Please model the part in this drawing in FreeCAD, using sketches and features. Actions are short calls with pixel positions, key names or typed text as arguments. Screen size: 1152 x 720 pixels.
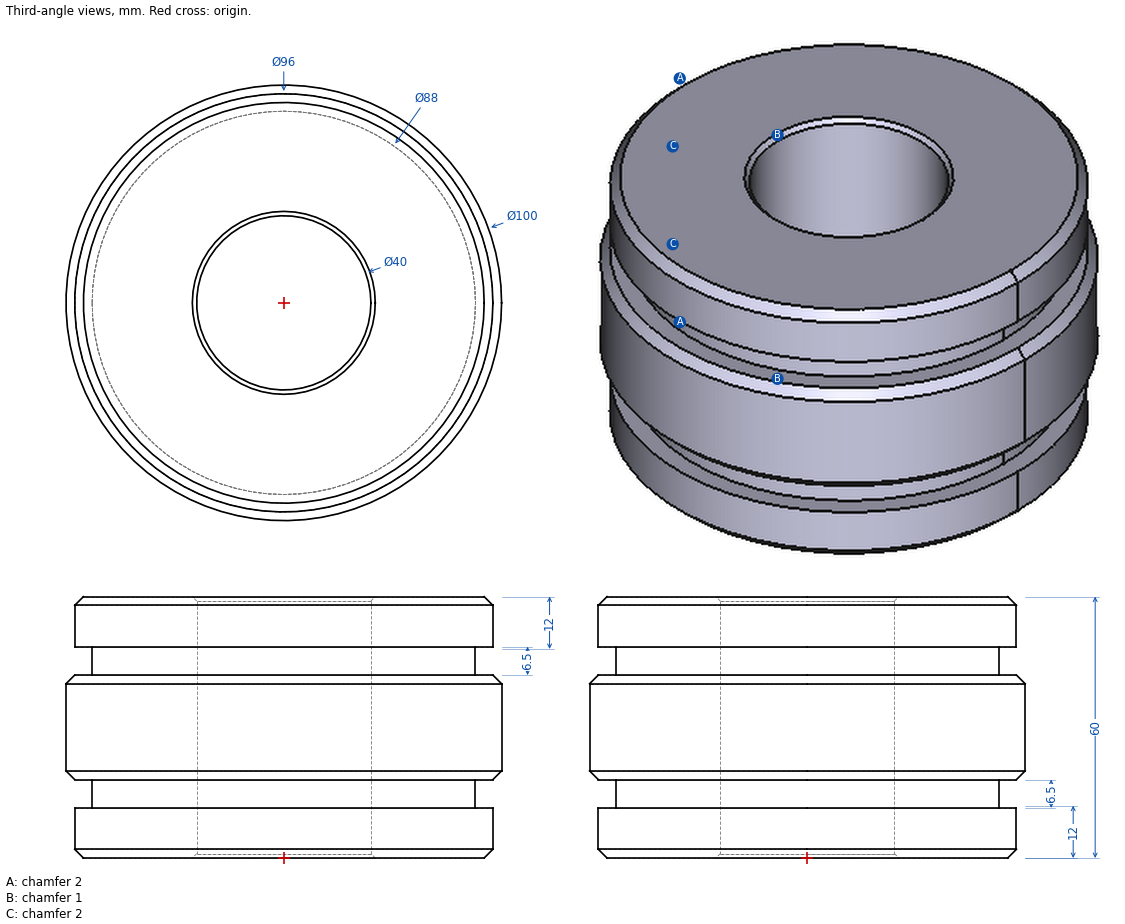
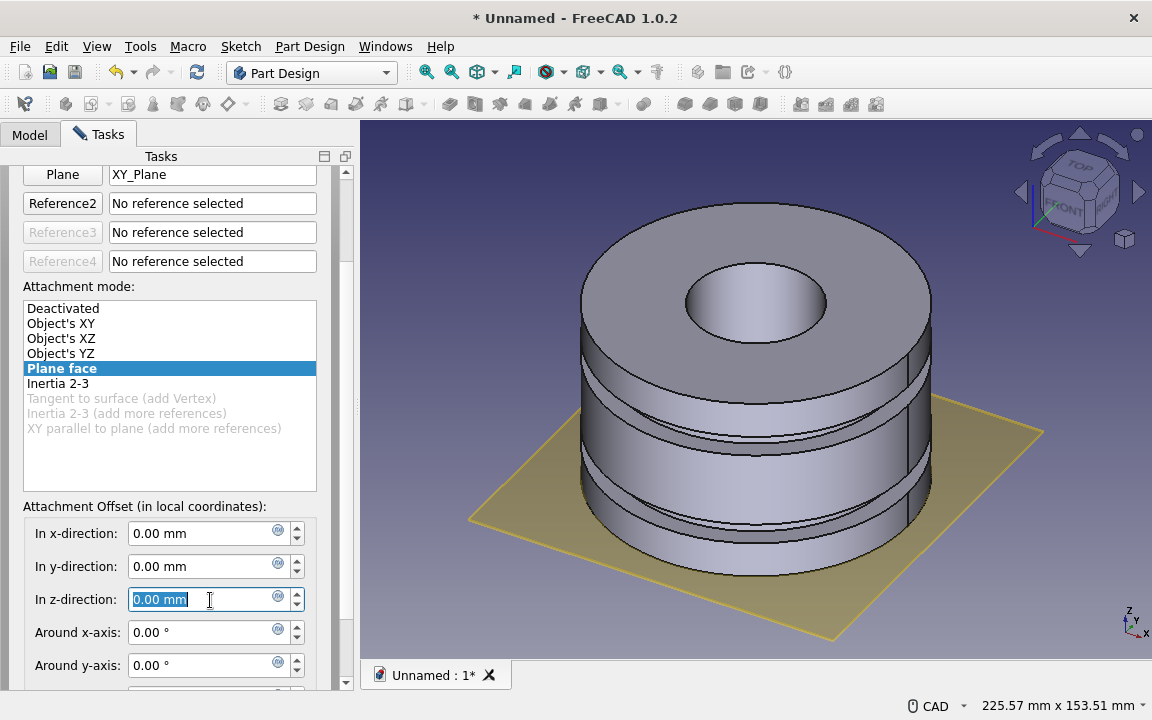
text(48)
key(Tab)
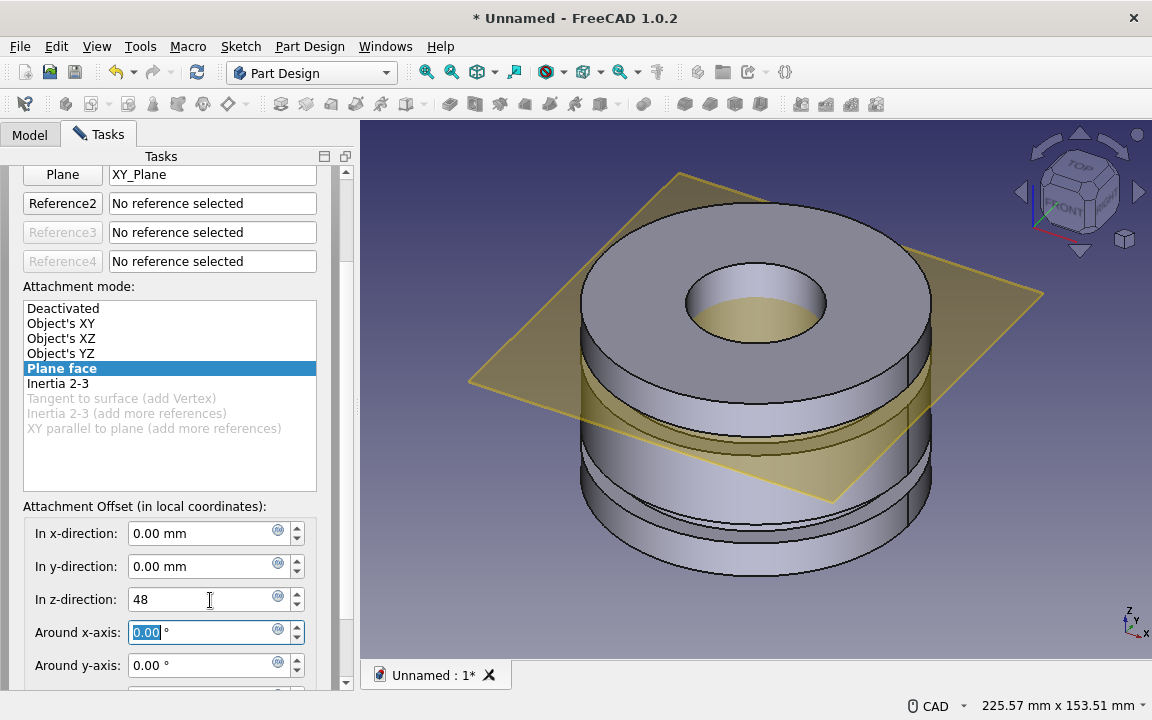
scroll(346, 428, up, 3)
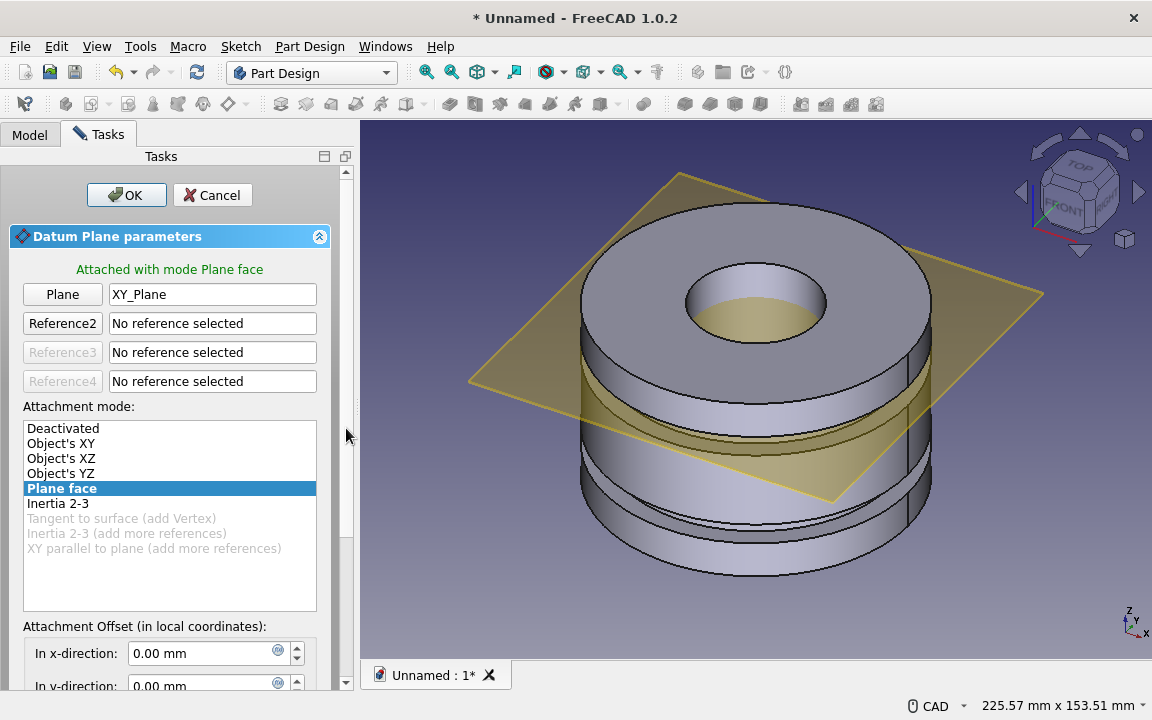
click(127, 195)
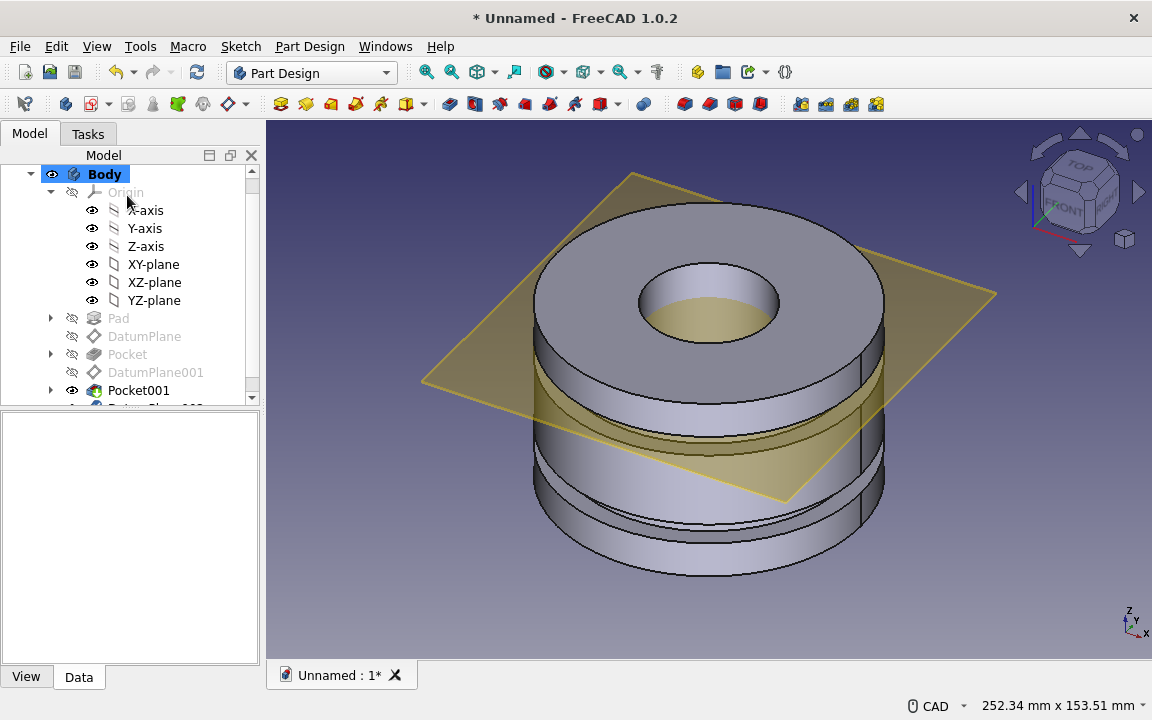
scroll(121, 278, down, 3)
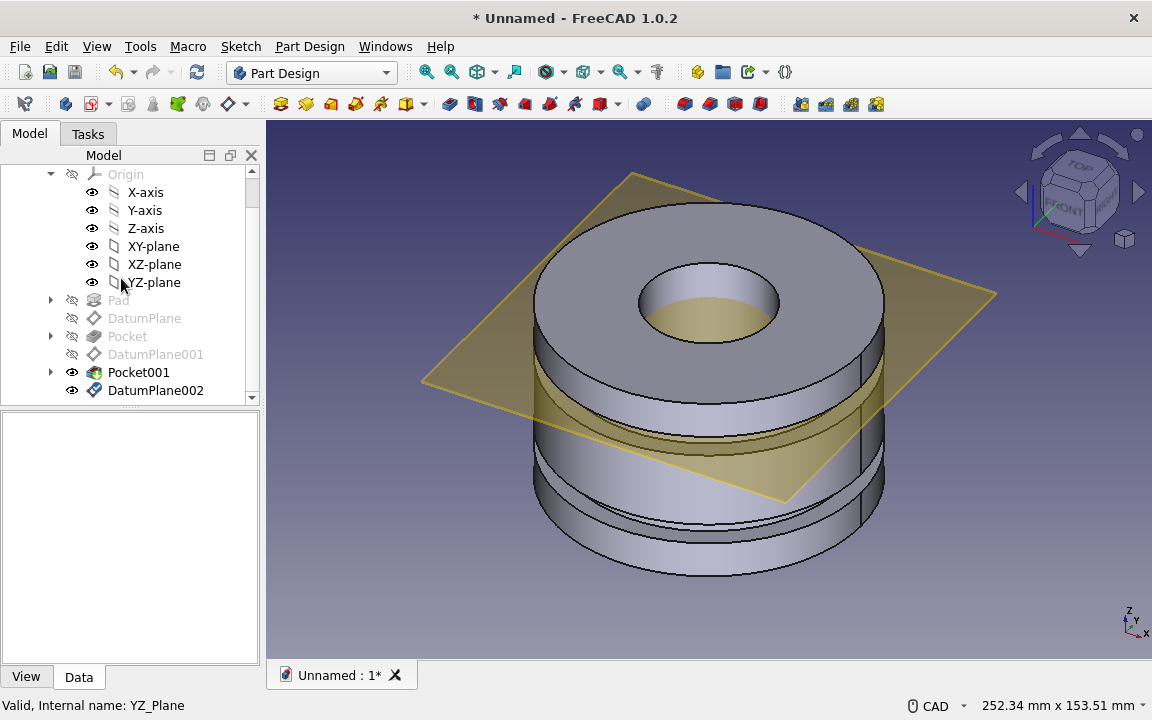
click(117, 390)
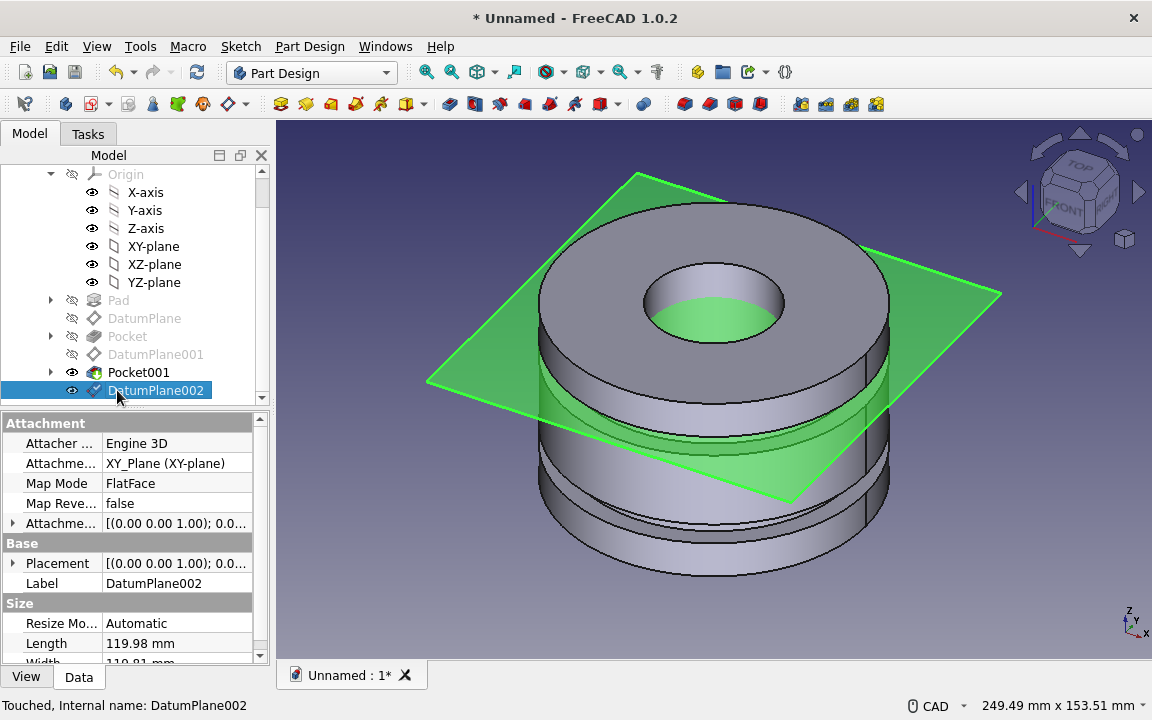
click(90, 104)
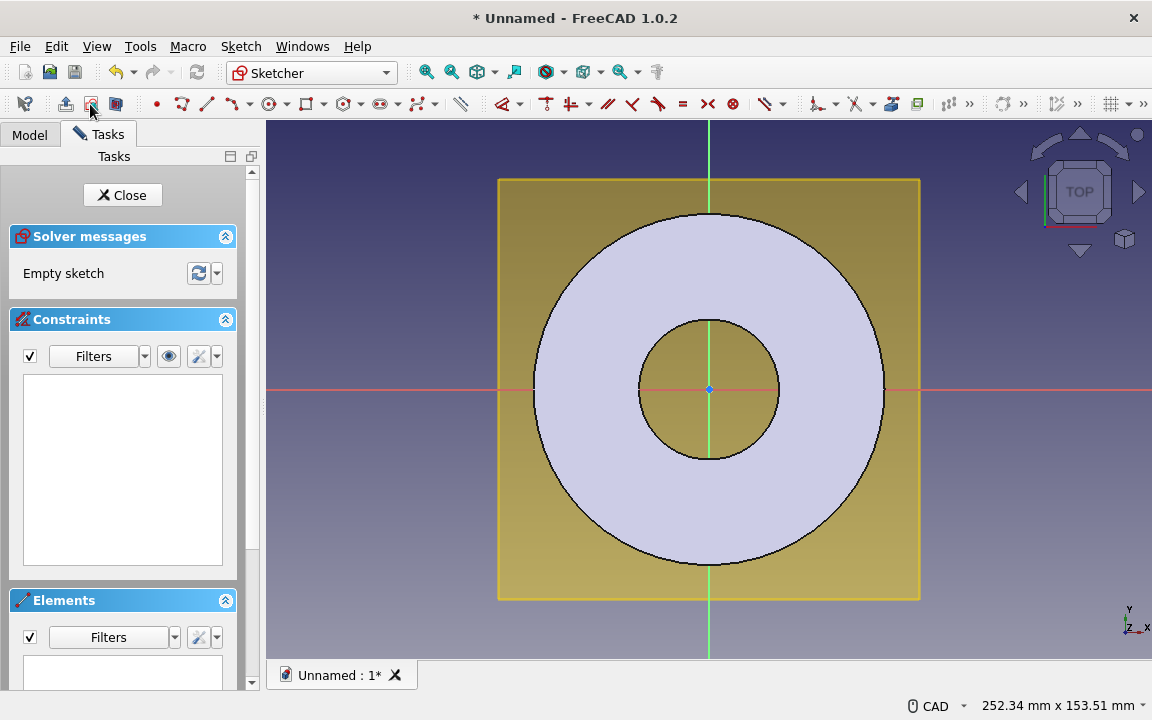
click(116, 104)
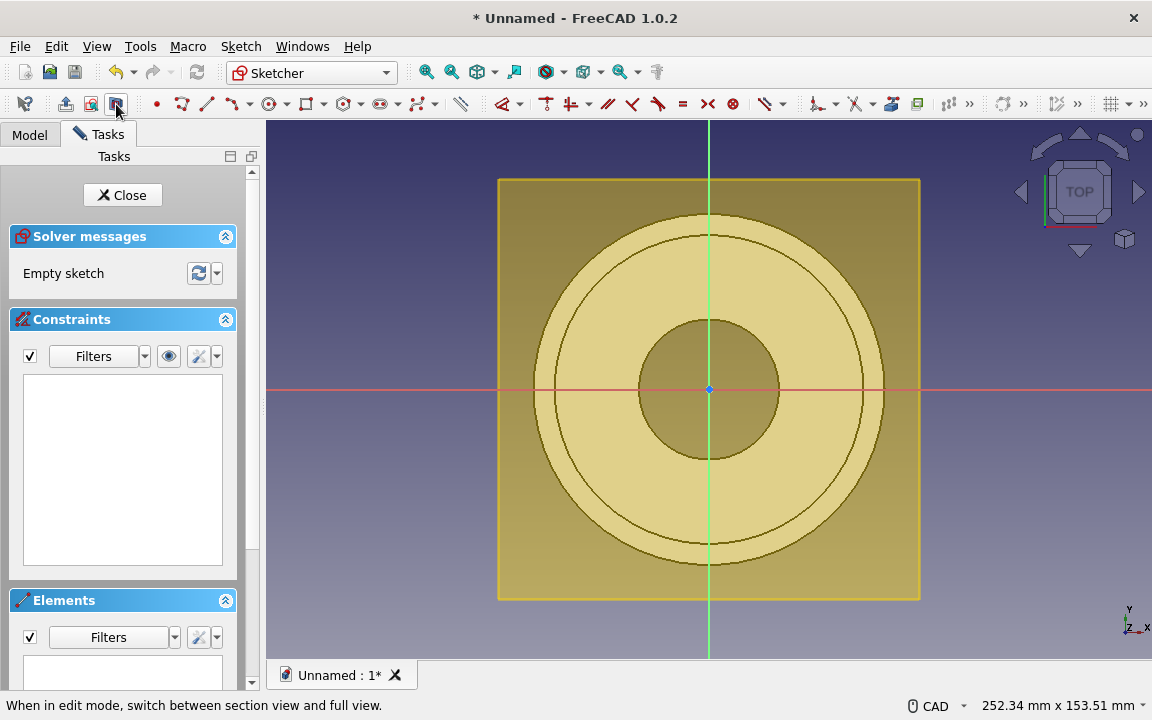
click(268, 104)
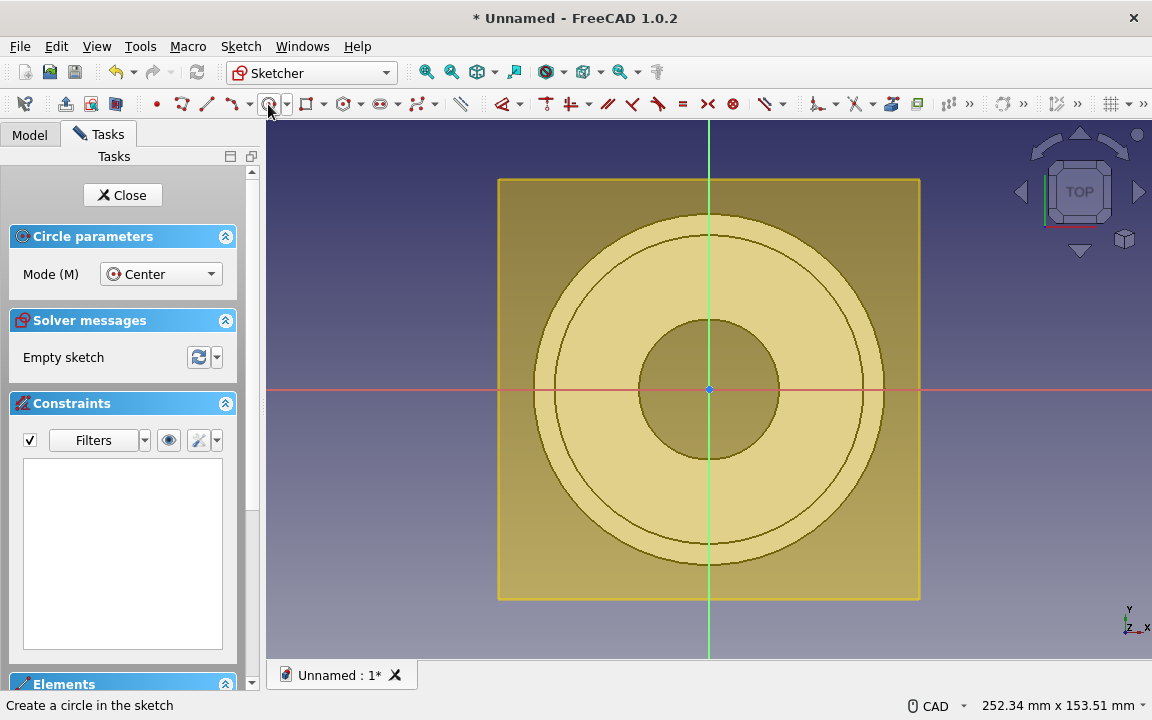
click(709, 390)
click(833, 265)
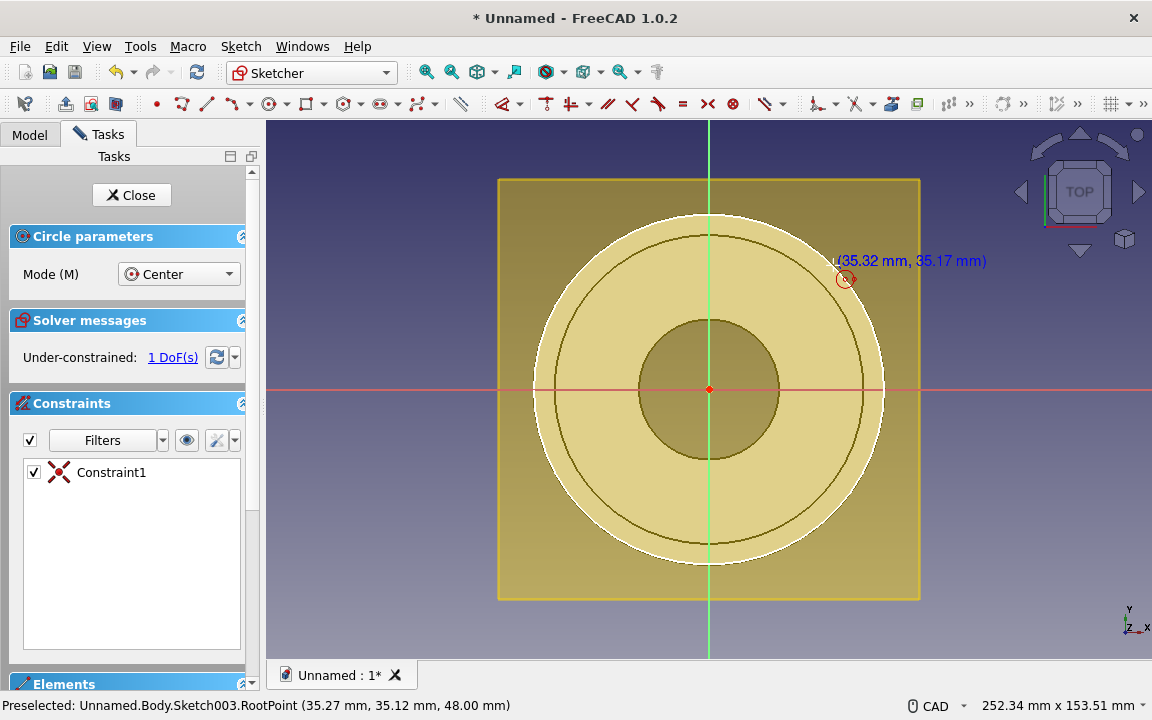
click(709, 390)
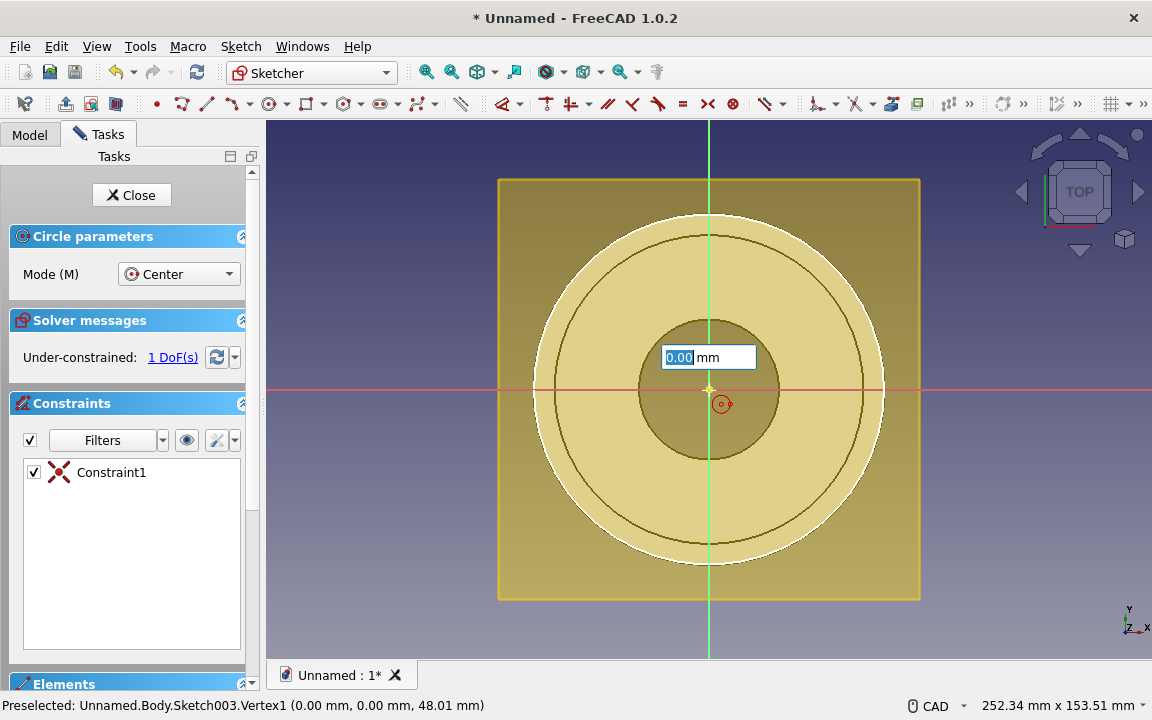
scroll(828, 509, up, 5)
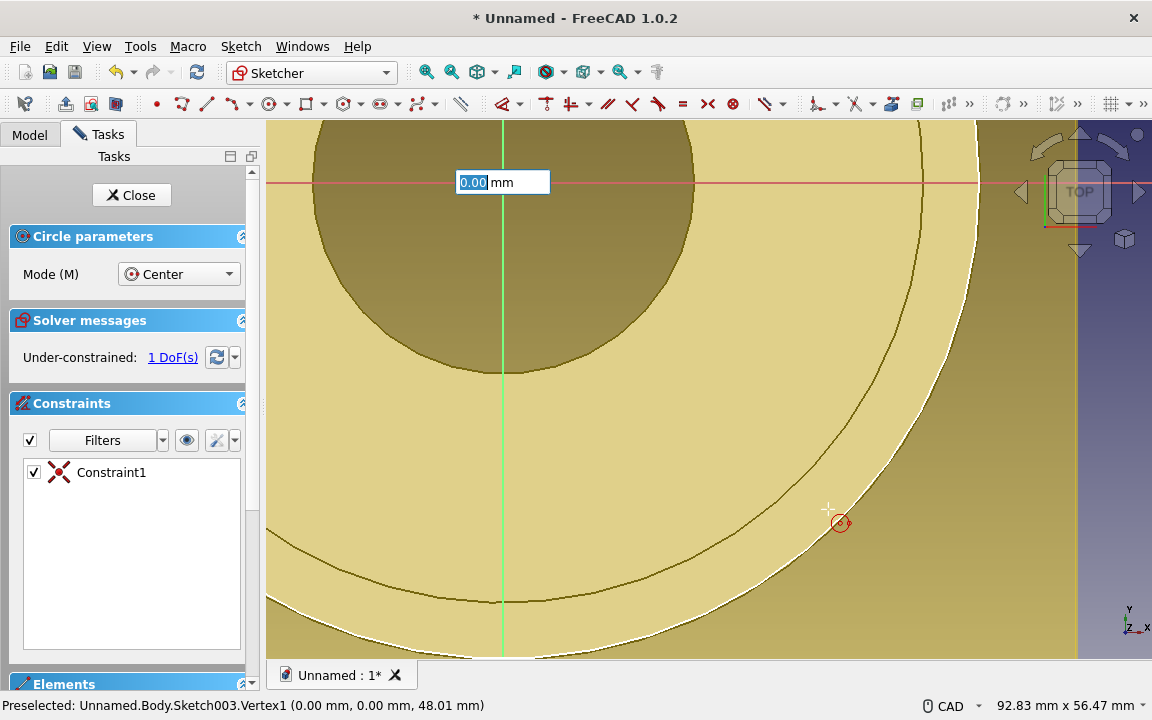
click(827, 507)
key(Escape)